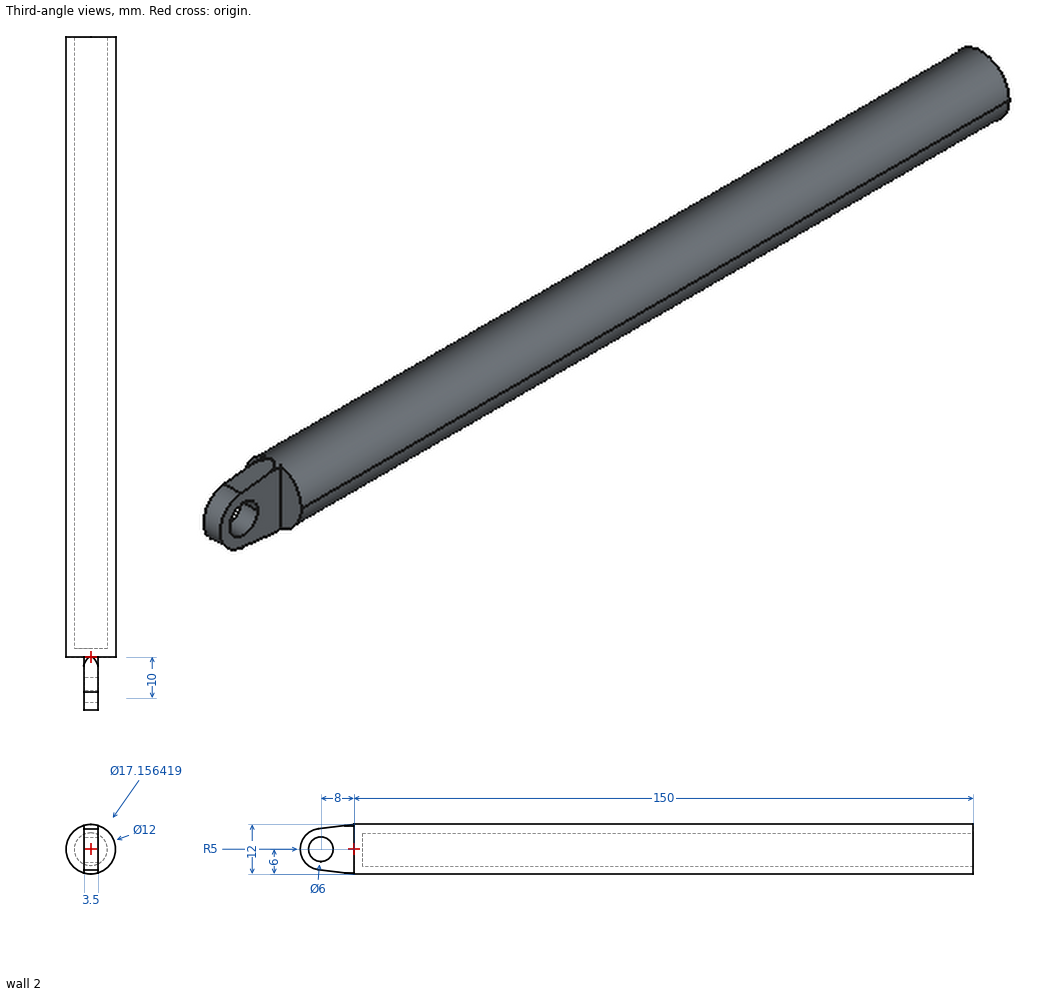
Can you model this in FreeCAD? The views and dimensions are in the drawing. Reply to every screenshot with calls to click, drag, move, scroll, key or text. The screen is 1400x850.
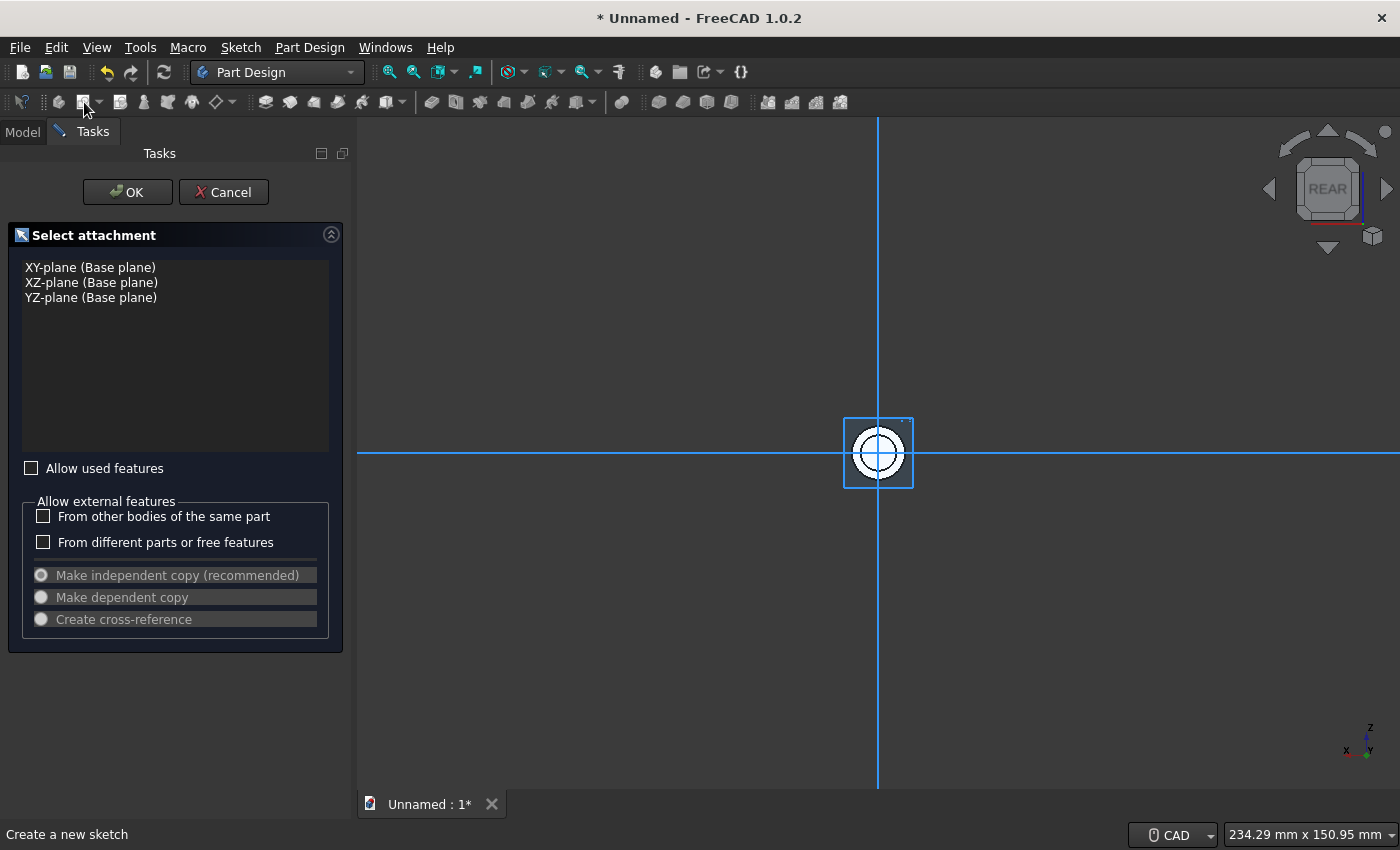
click(82, 298)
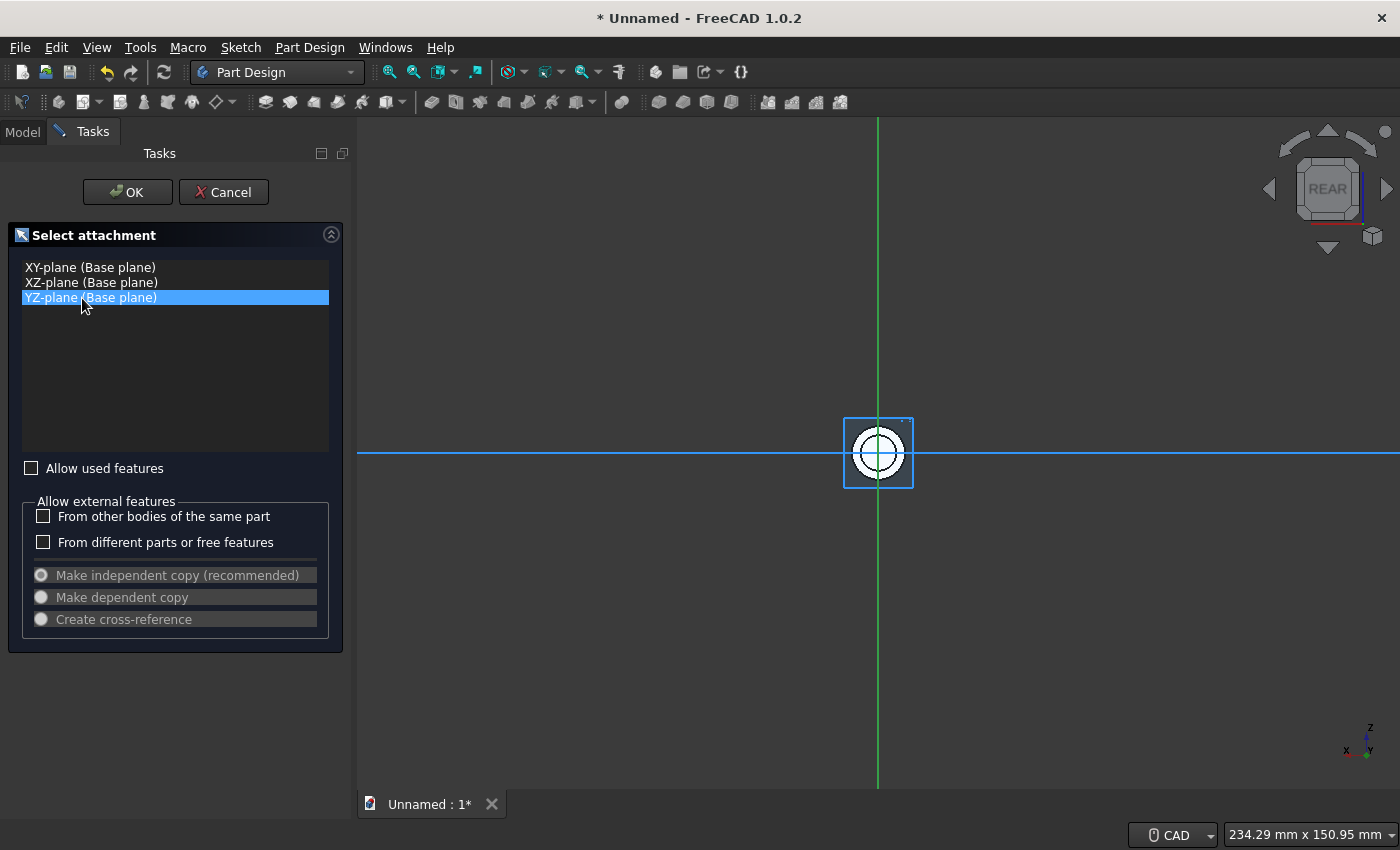
click(128, 192)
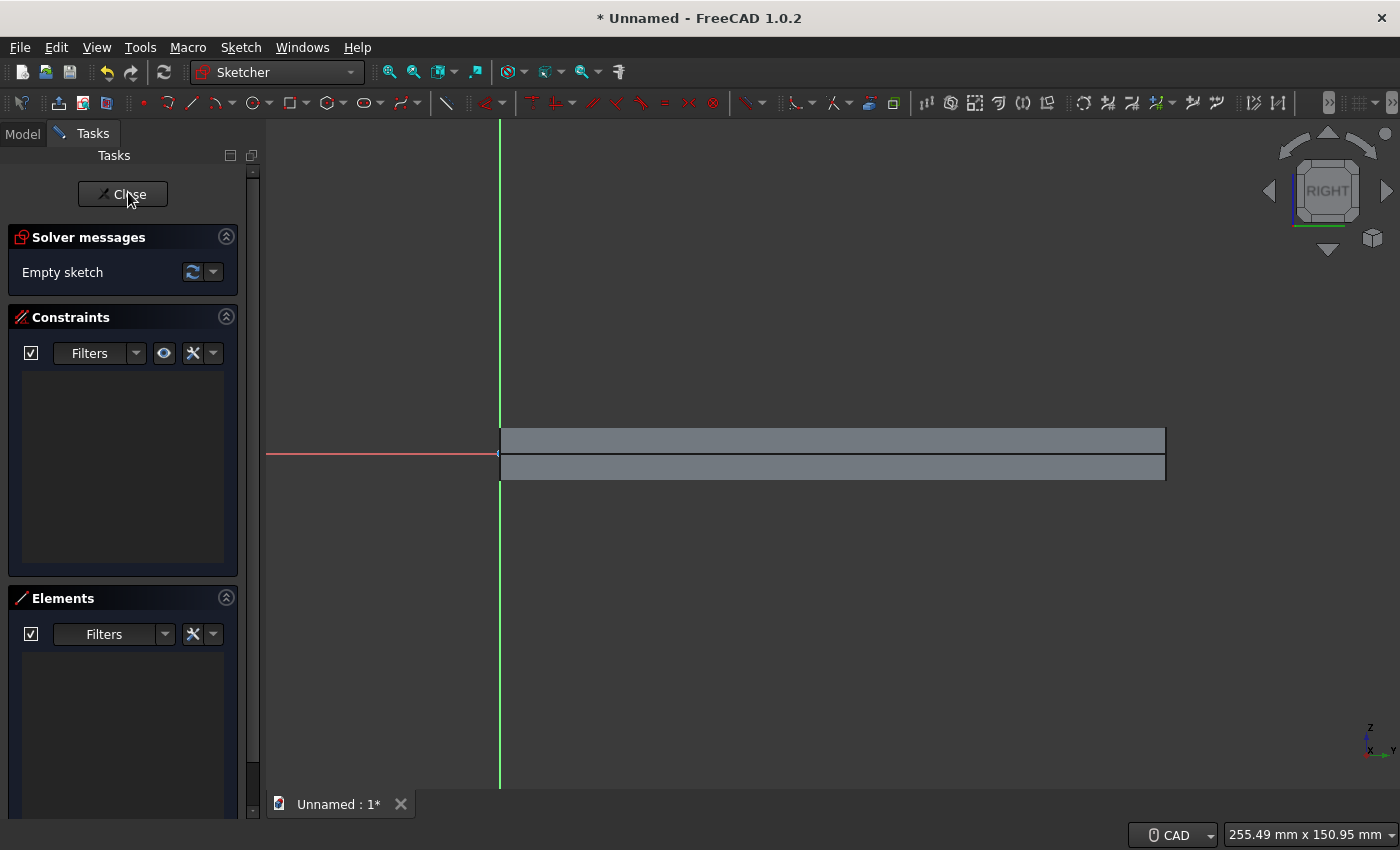
click(108, 104)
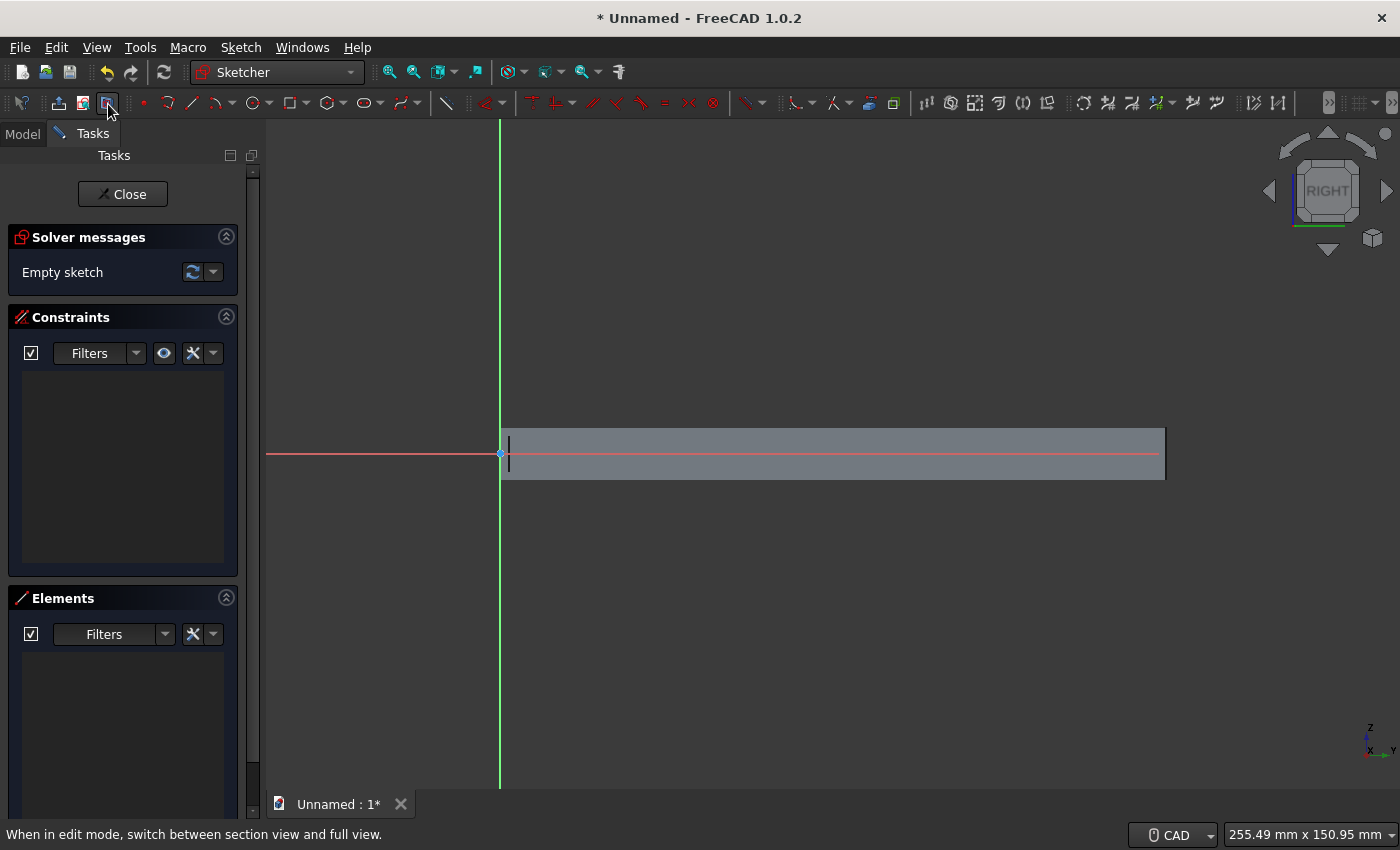
scroll(425, 454, up, 10)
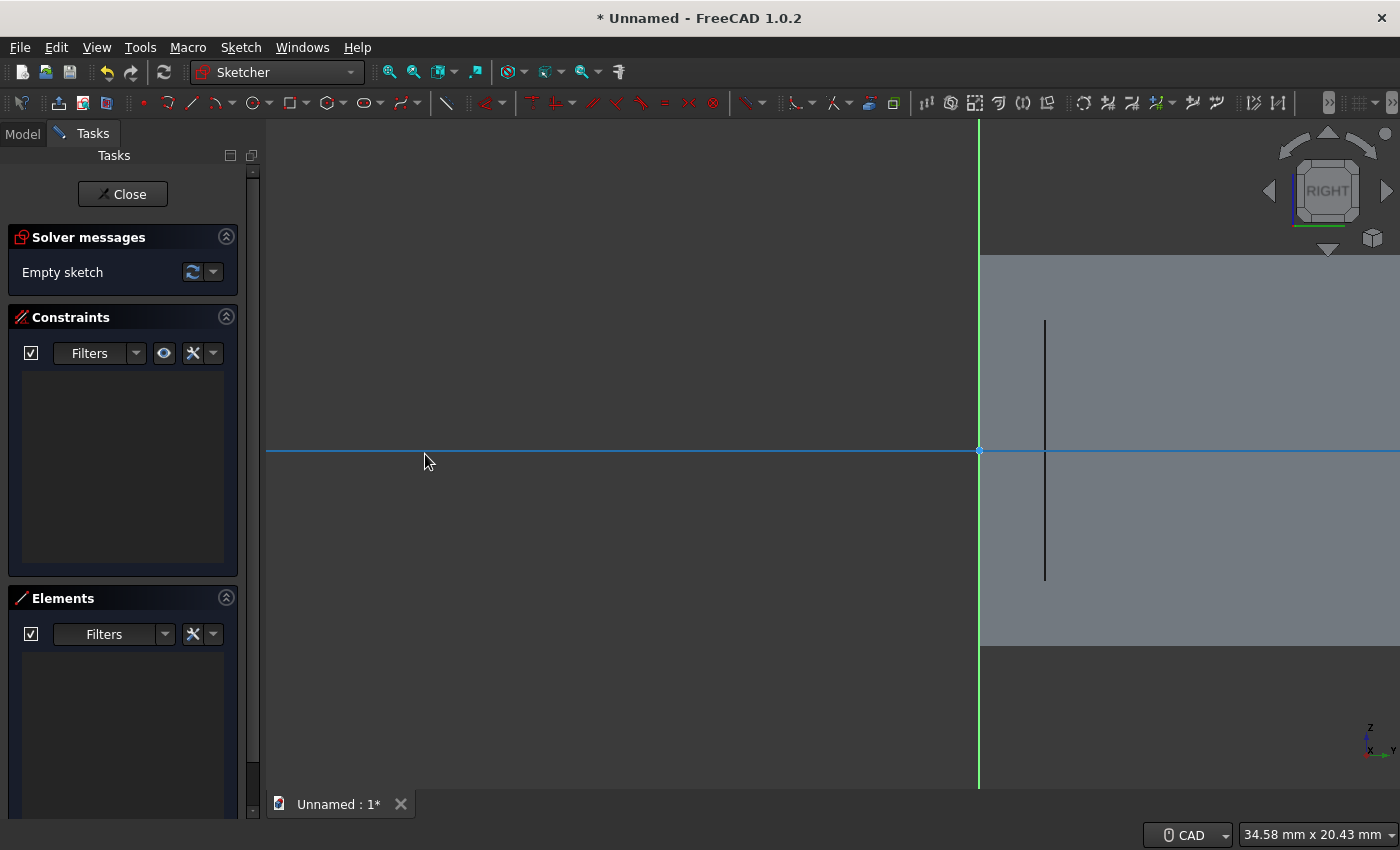
click(168, 104)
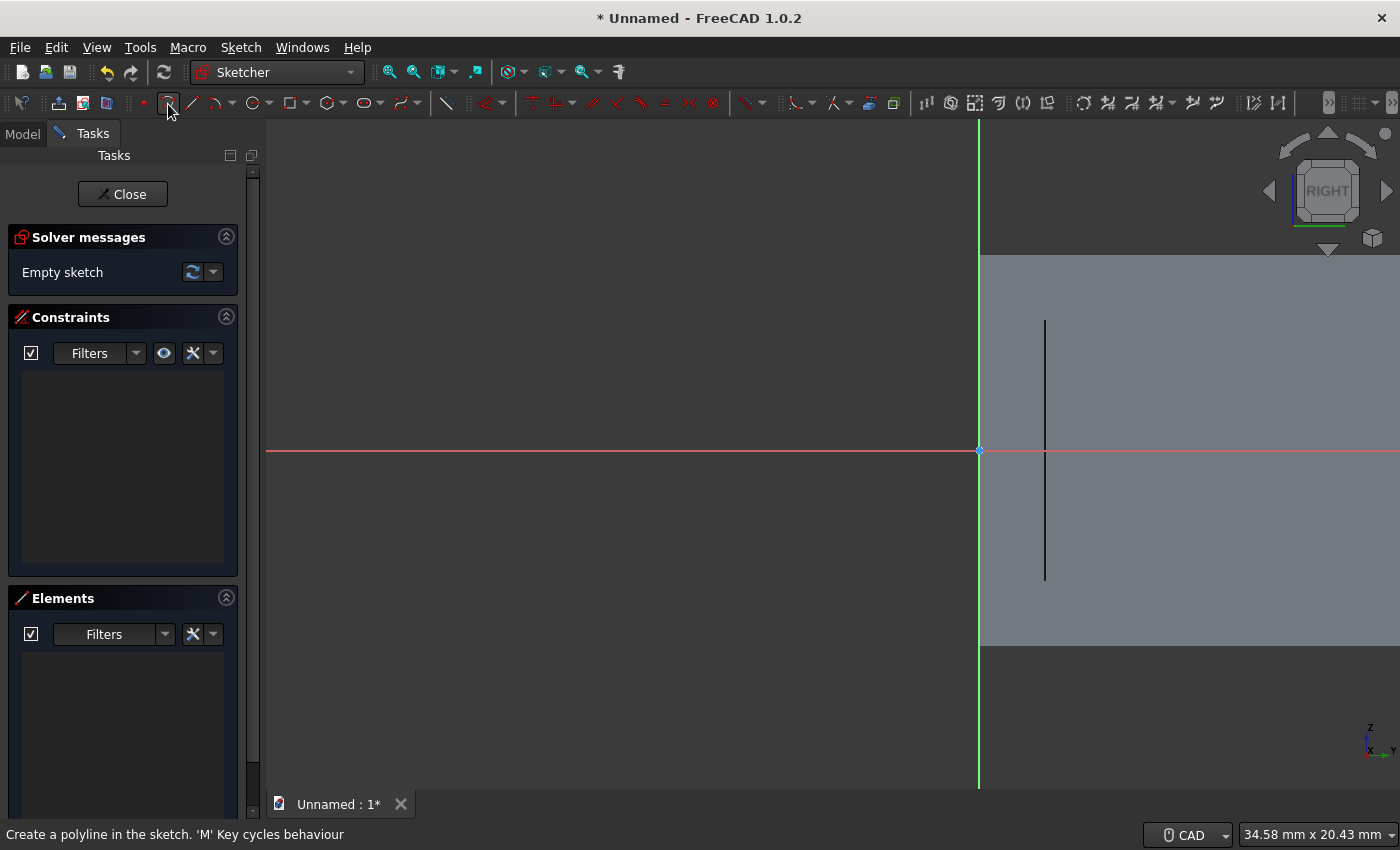
click(697, 614)
click(979, 648)
click(970, 254)
click(697, 288)
right_click(697, 288)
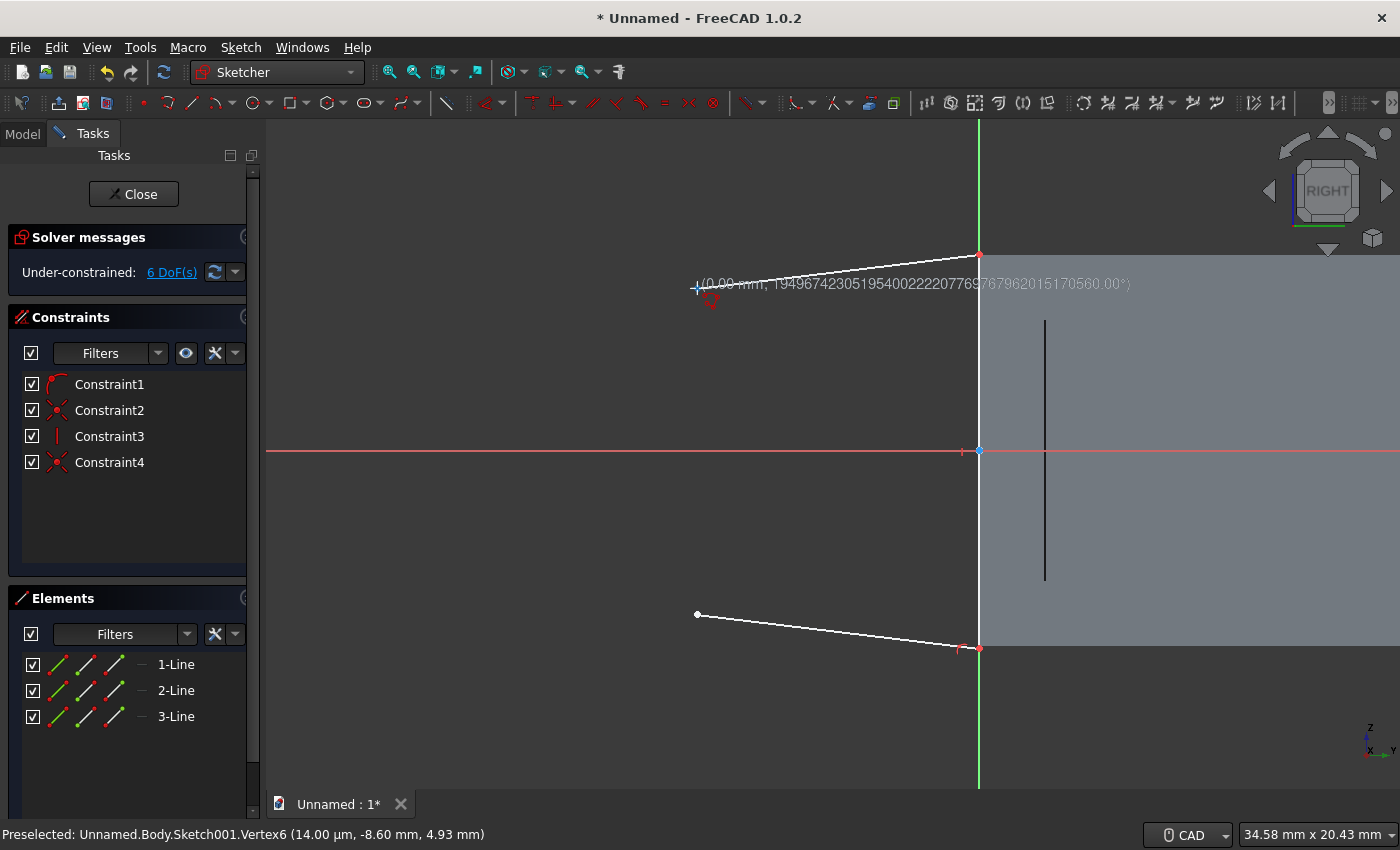
click(234, 104)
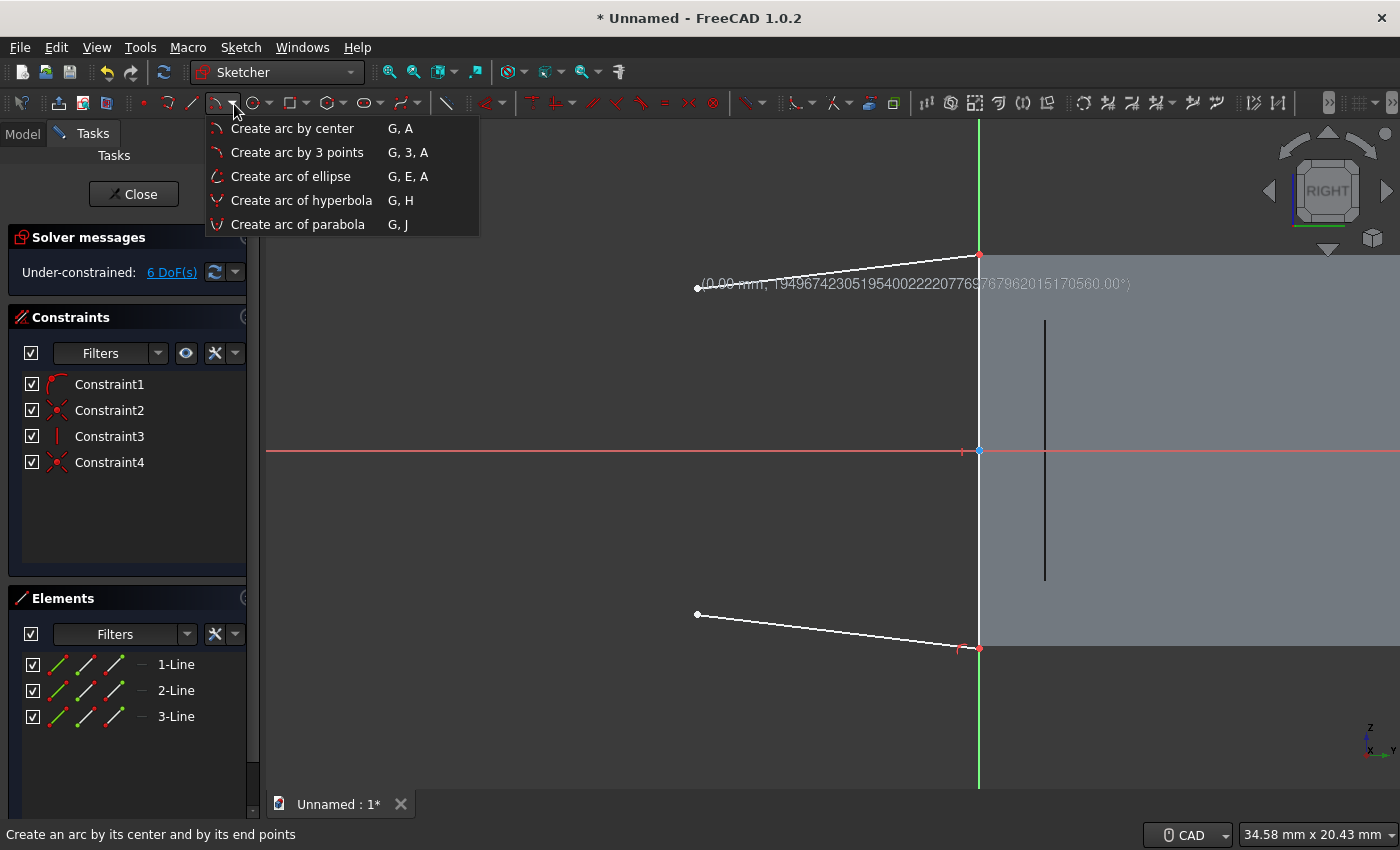
click(342, 152)